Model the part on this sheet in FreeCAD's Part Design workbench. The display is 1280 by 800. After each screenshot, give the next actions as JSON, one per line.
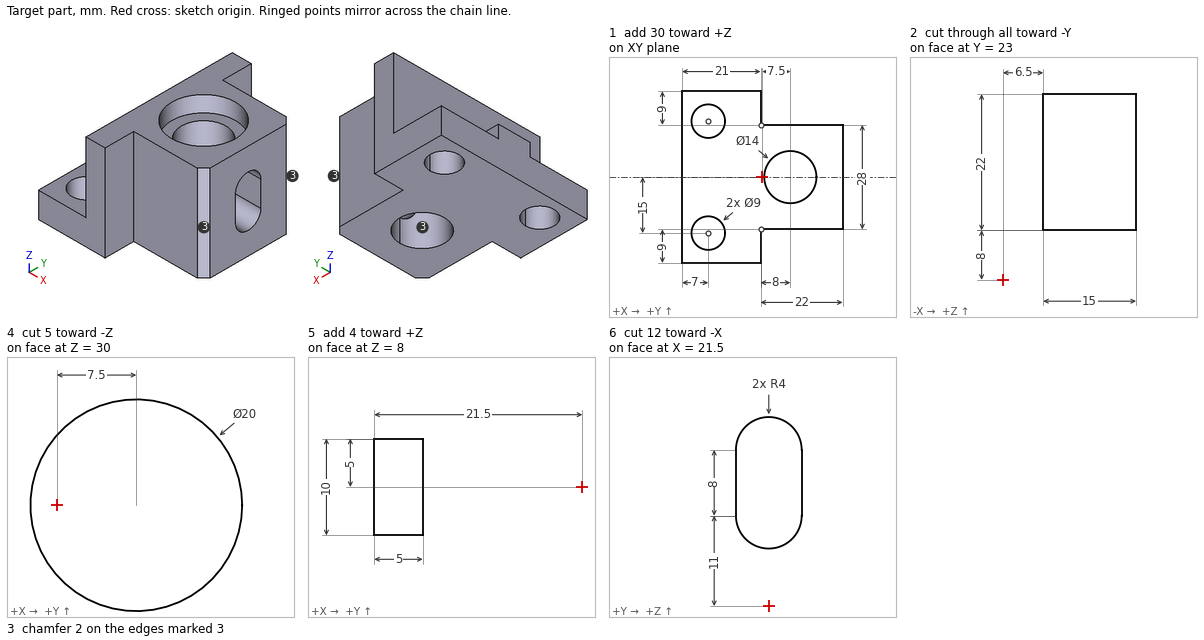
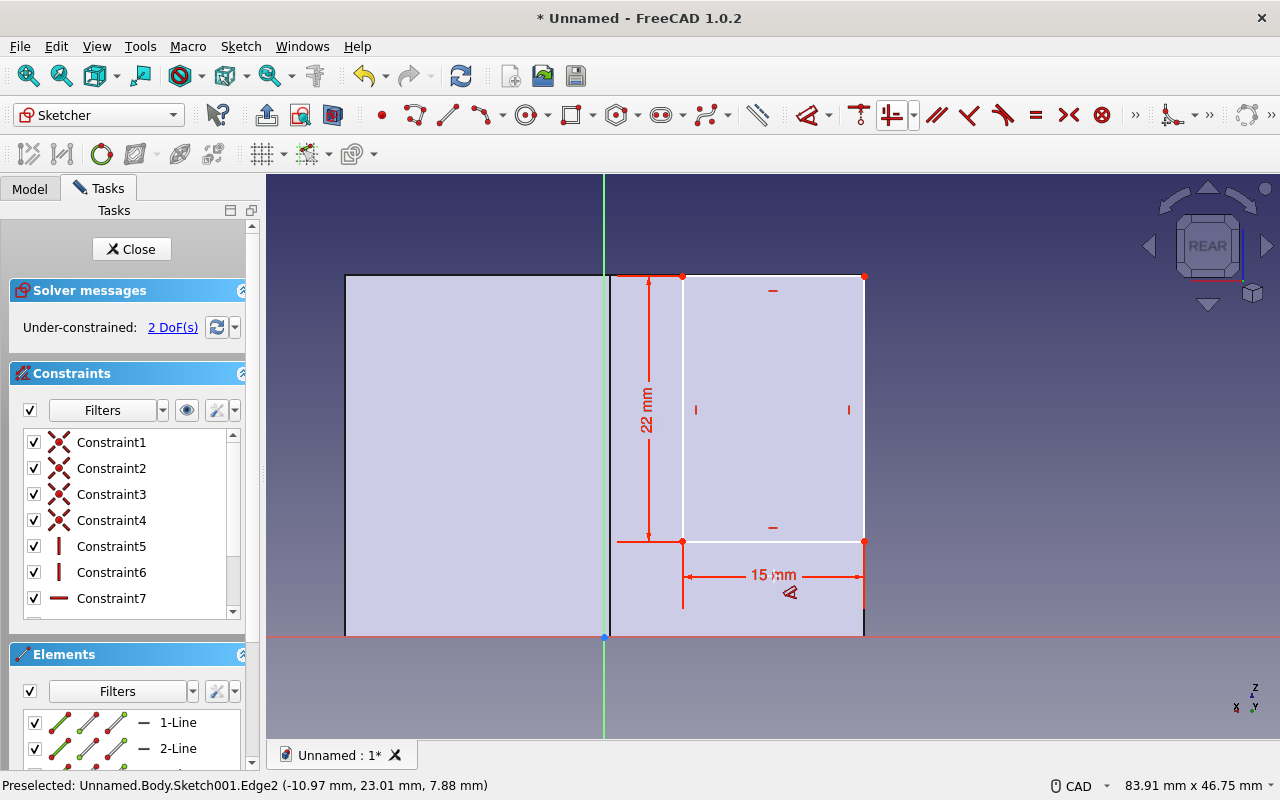
{"action": "left_click", "coordinate": [683, 542]}
{"action": "left_click", "coordinate": [570, 590]}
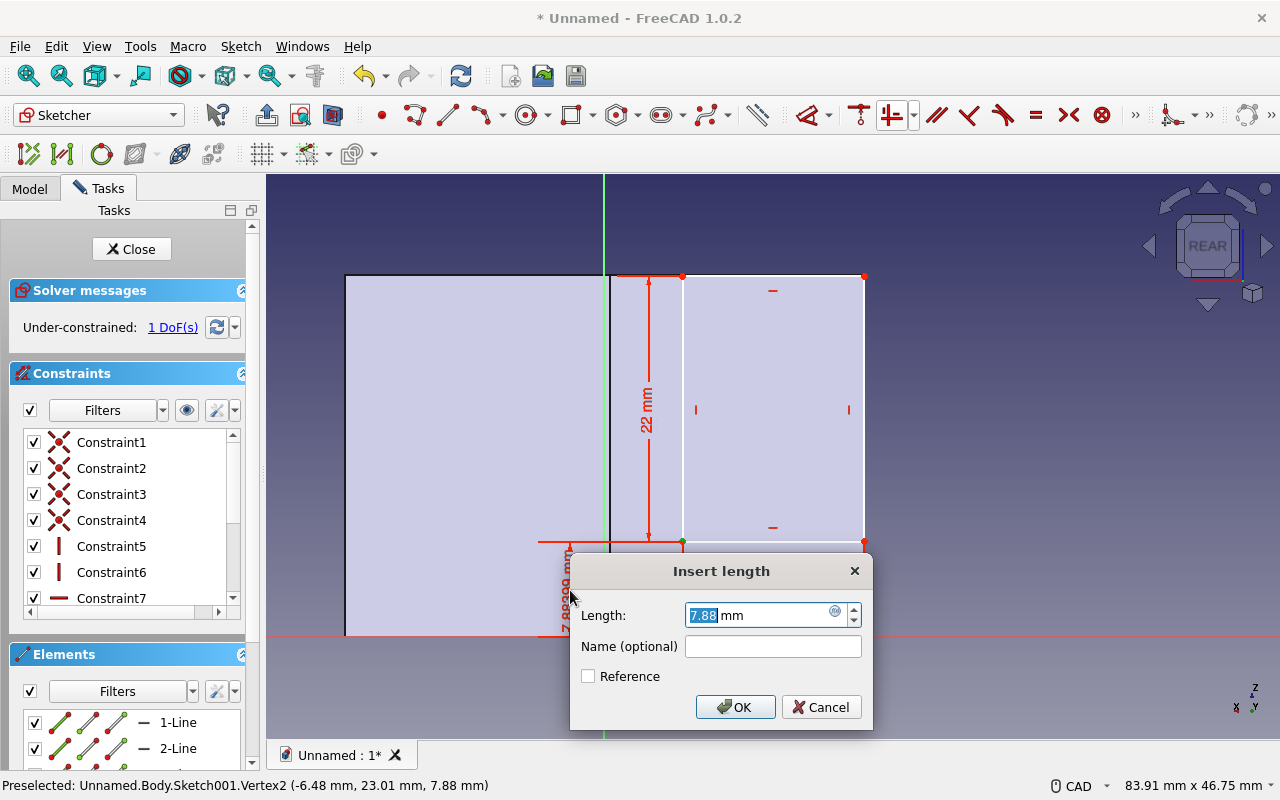
{"action": "type", "text": "8"}
{"action": "key", "text": "Return"}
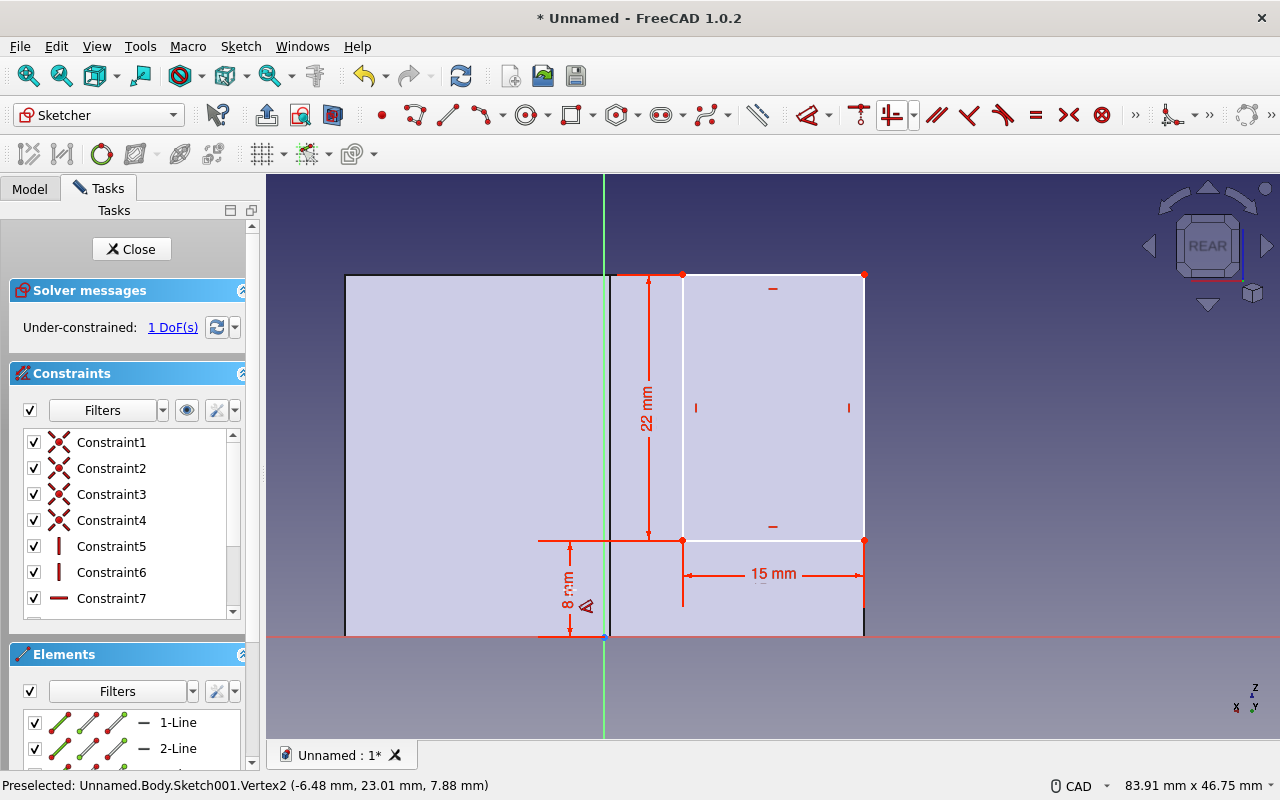
{"action": "left_click", "coordinate": [683, 275]}
{"action": "left_click", "coordinate": [644, 671]}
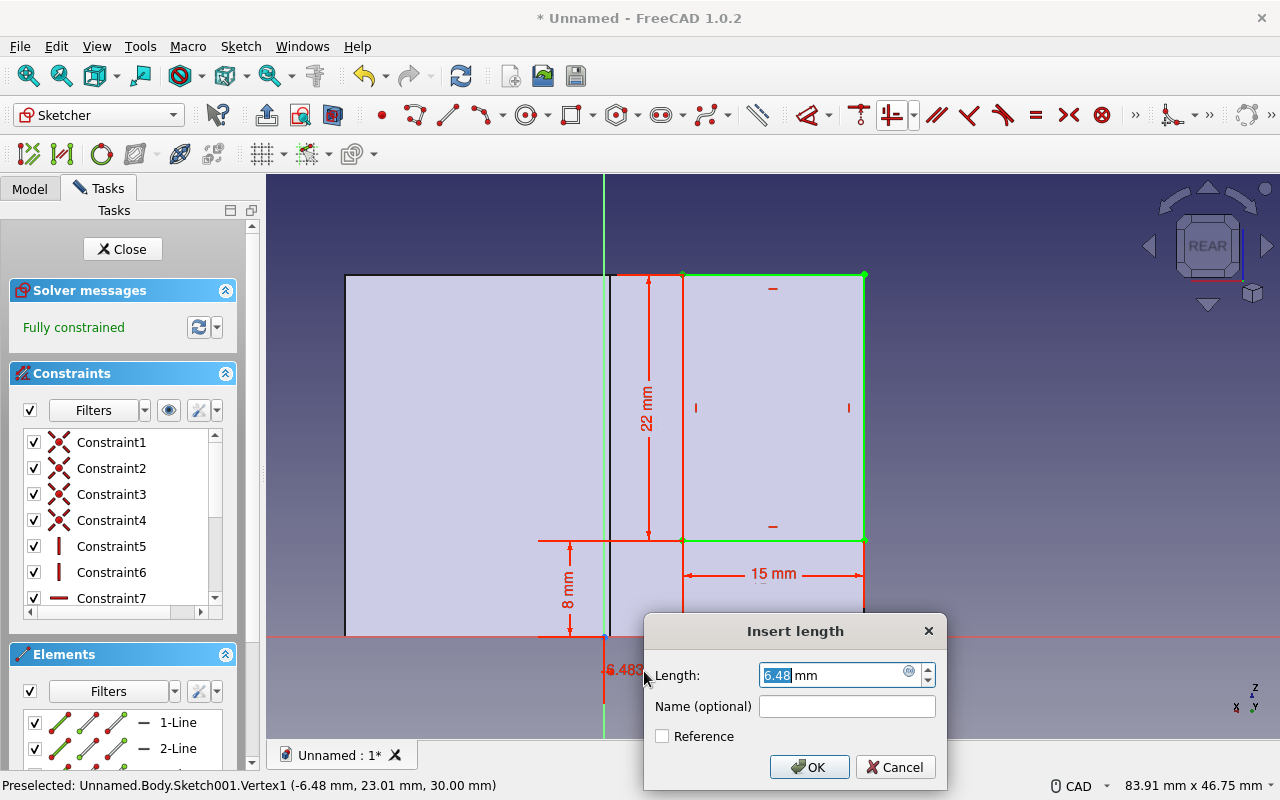
{"action": "type", "text": "6.5"}
{"action": "key", "text": "Return"}
{"action": "key", "text": "Escape"}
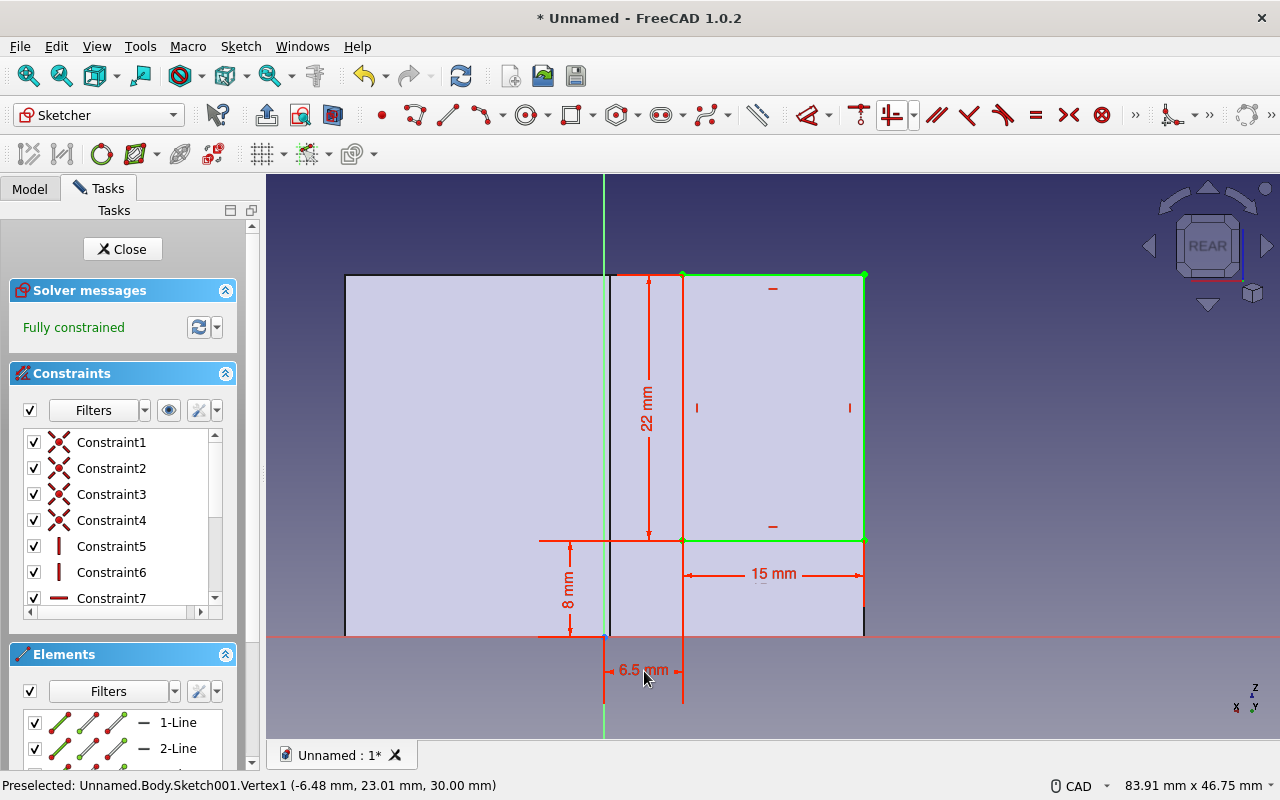
{"action": "left_click", "coordinate": [123, 249]}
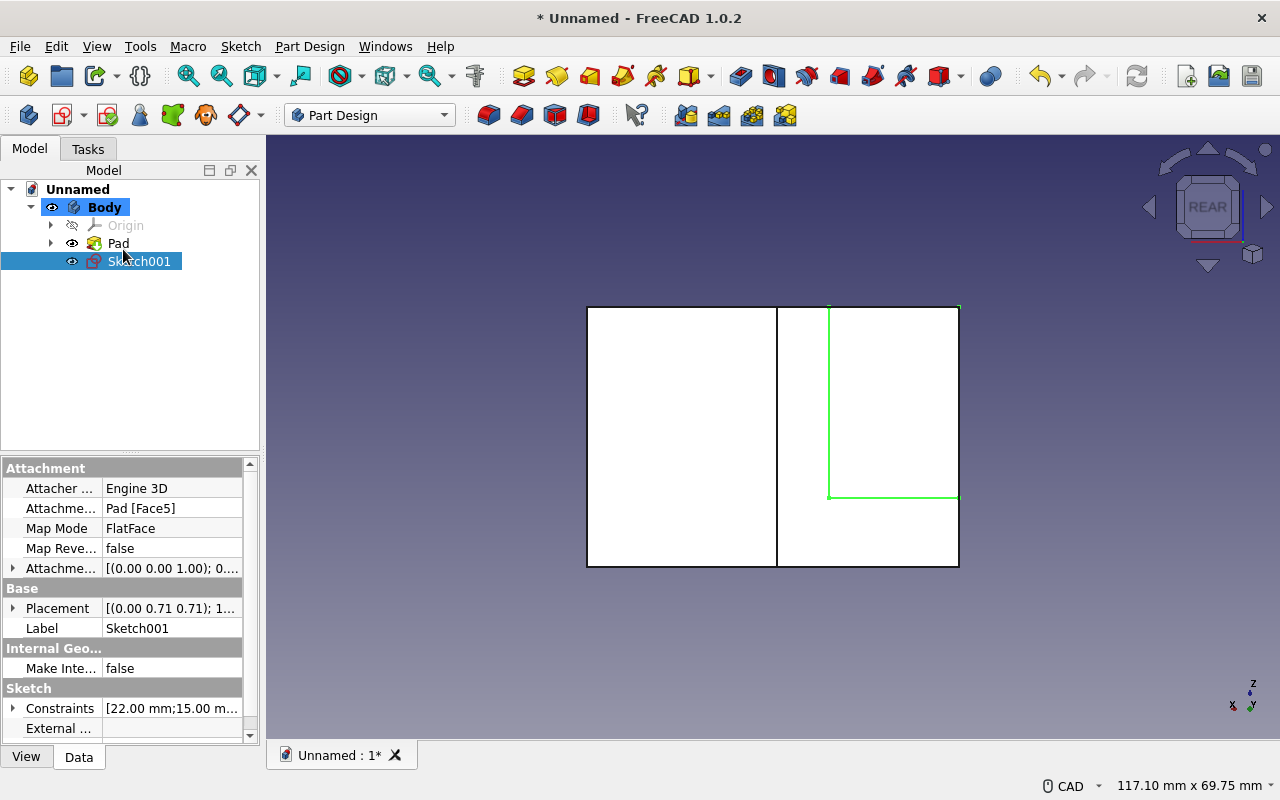
{"action": "left_click", "coordinate": [741, 76]}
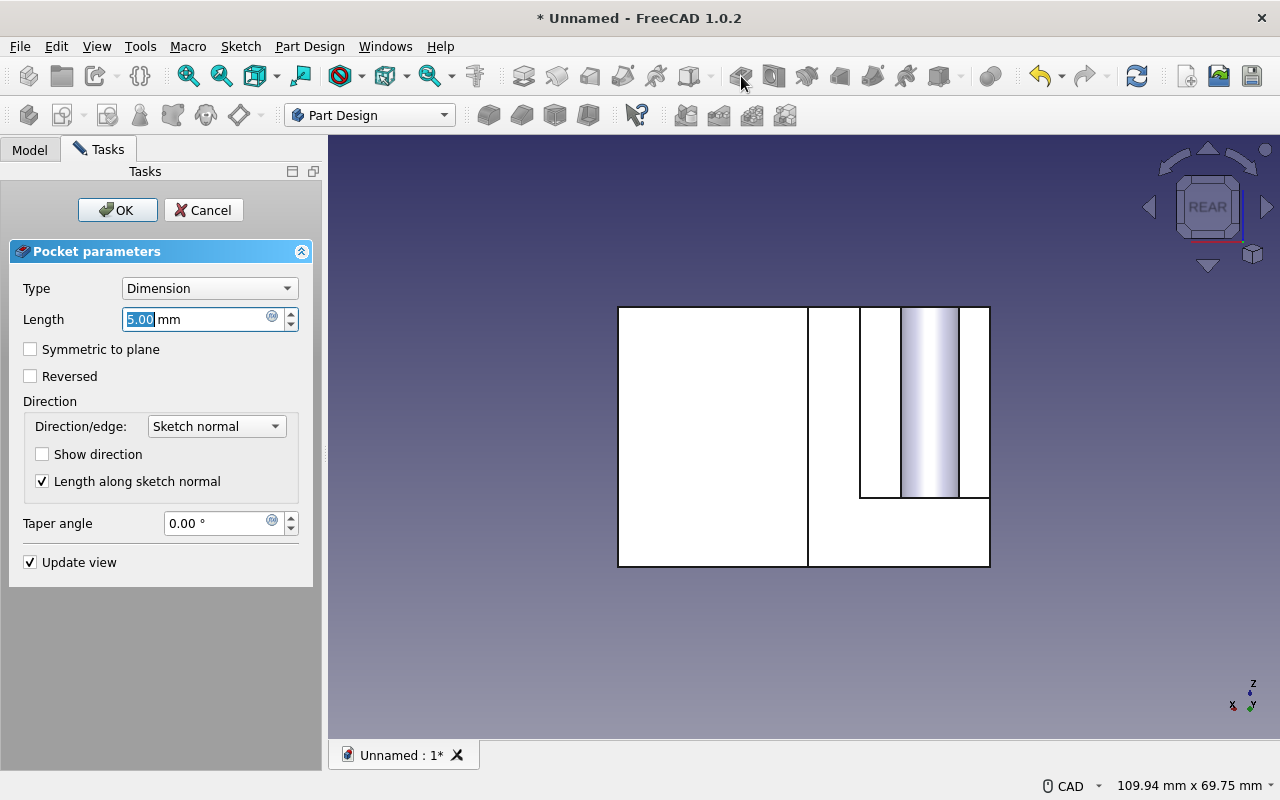
{"action": "left_click", "coordinate": [210, 288]}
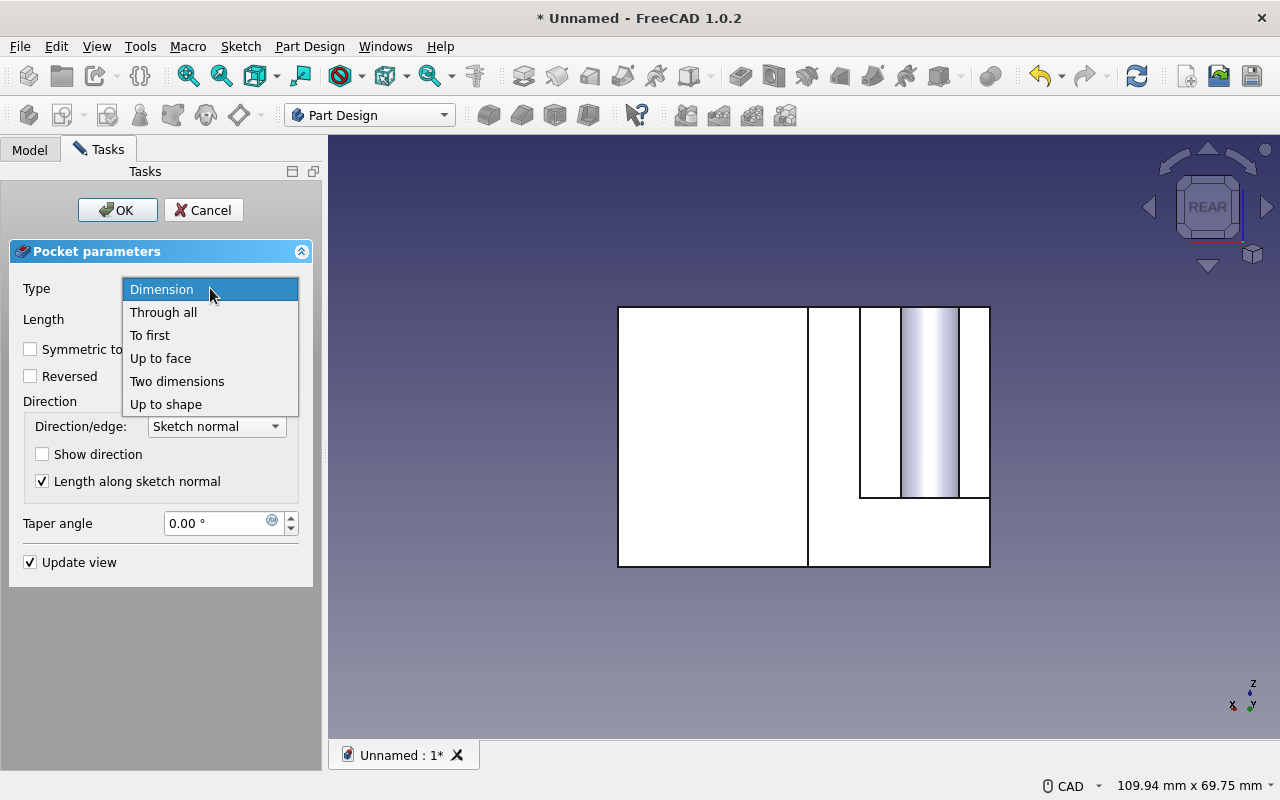
{"action": "left_click", "coordinate": [208, 312]}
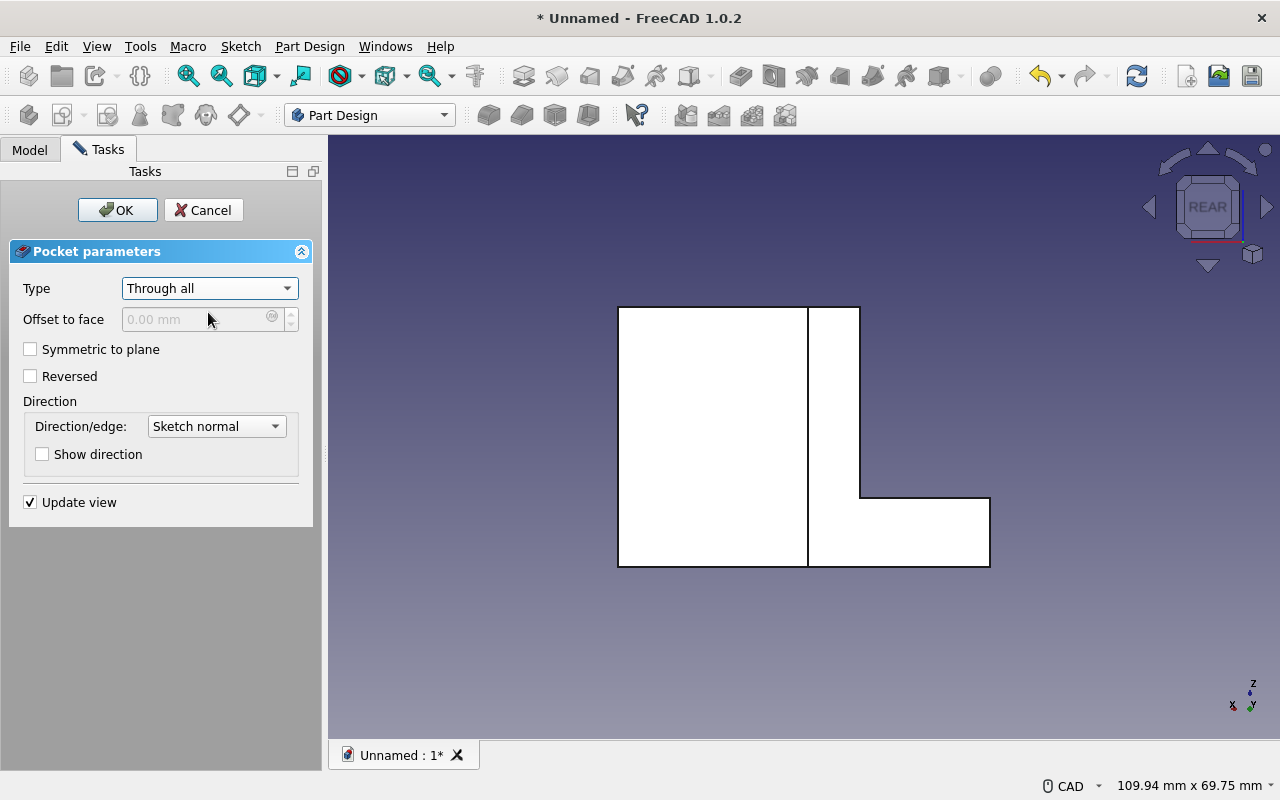
{"action": "left_click", "coordinate": [118, 210]}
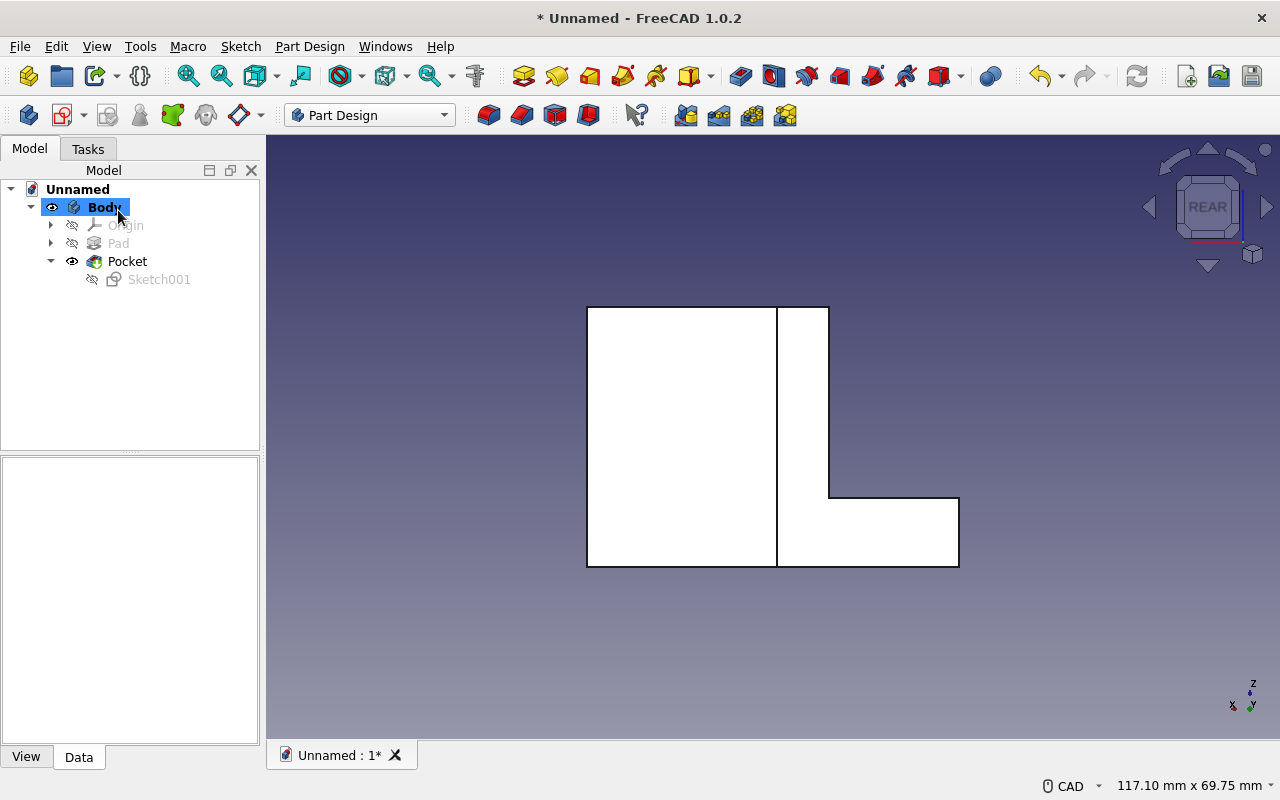
{"action": "key", "text": "v f"}